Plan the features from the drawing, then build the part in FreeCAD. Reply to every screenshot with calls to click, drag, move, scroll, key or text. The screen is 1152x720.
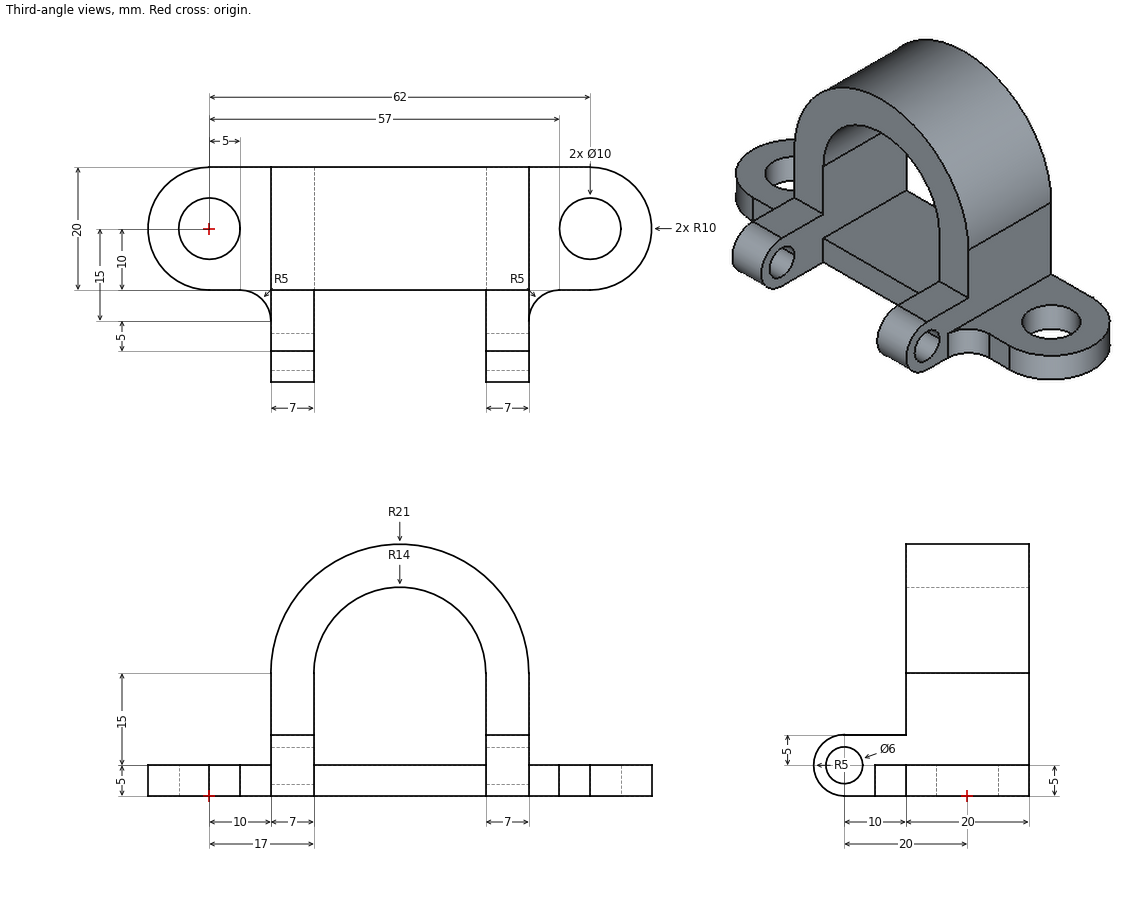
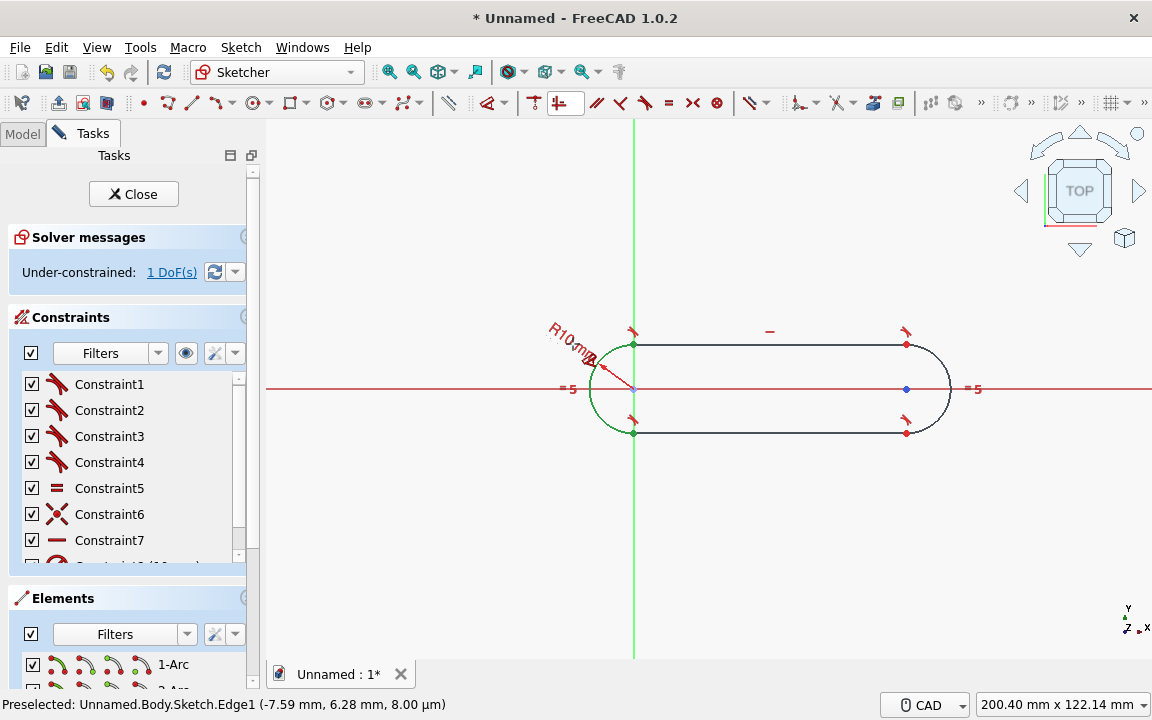
click(716, 345)
click(770, 311)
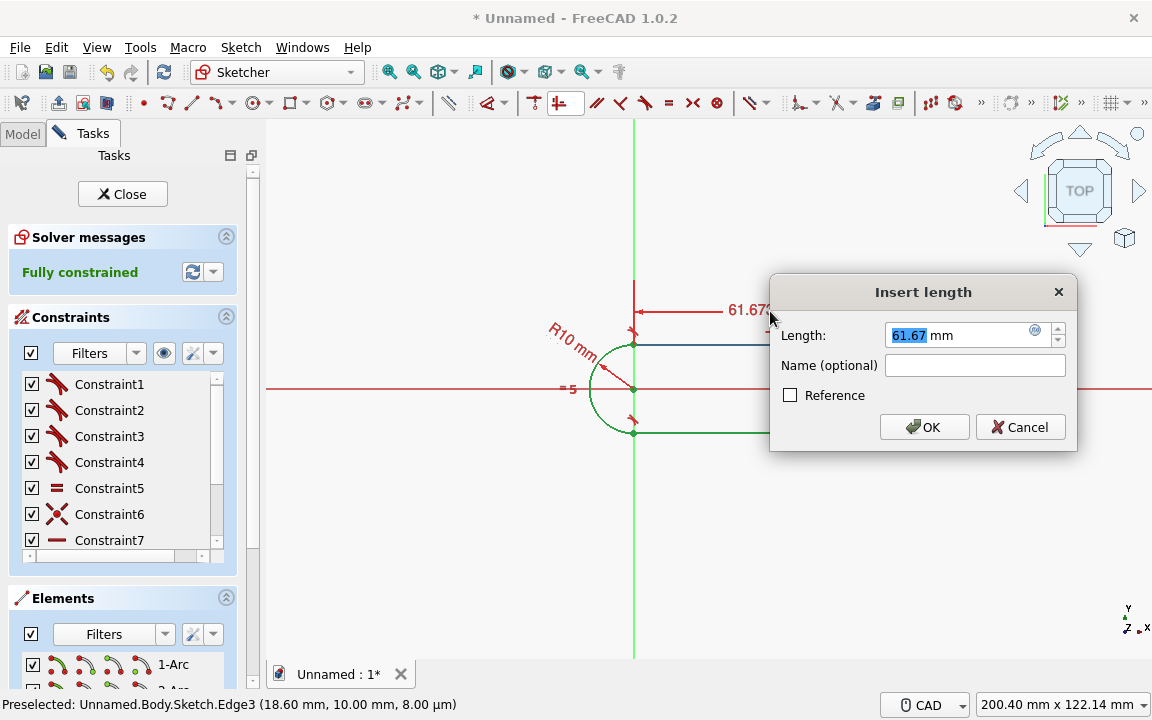
text(62)
key(Return)
key(Escape)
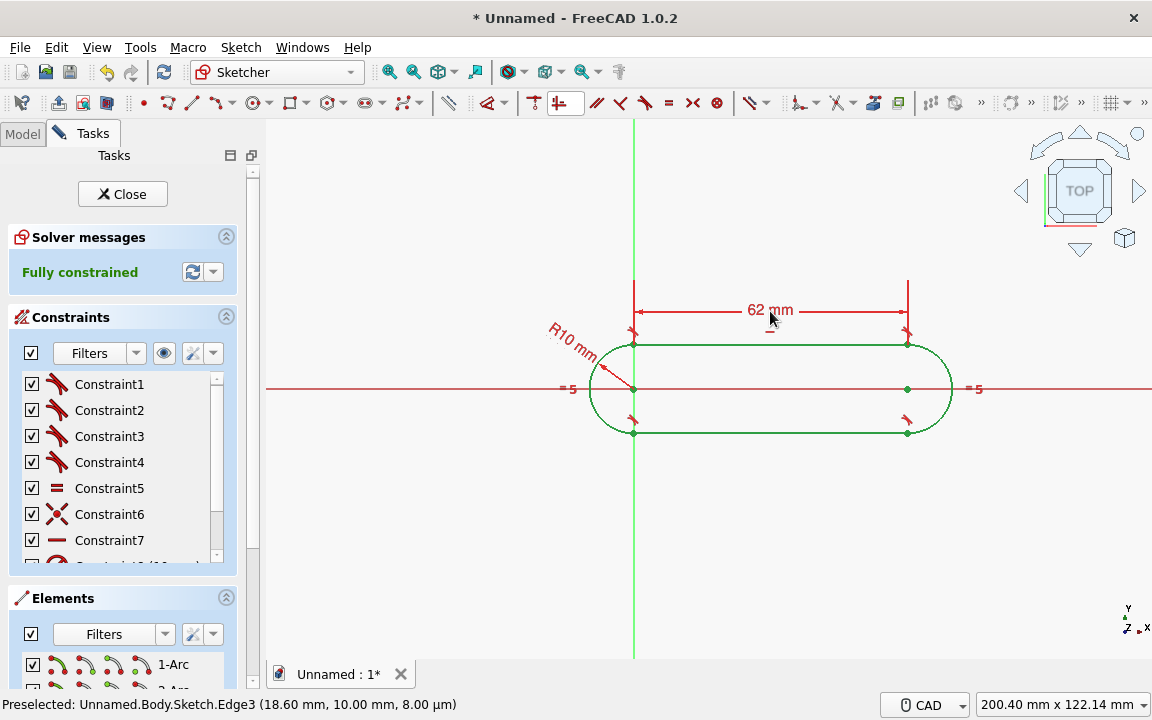
click(123, 194)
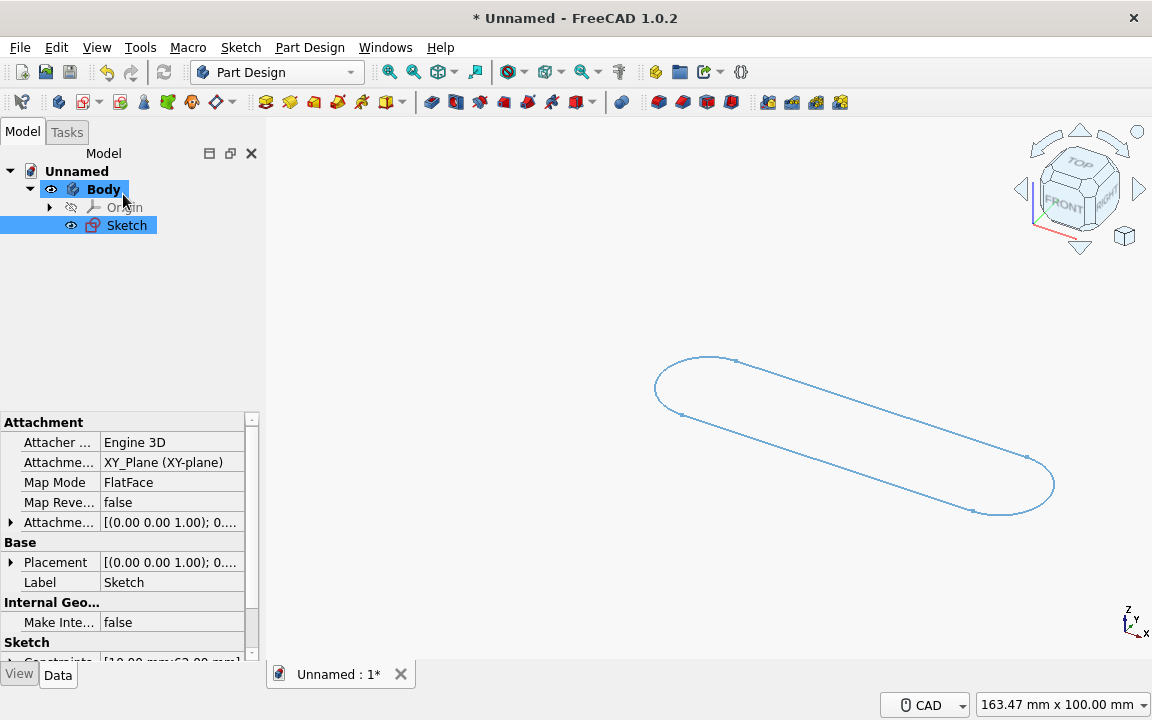
click(266, 102)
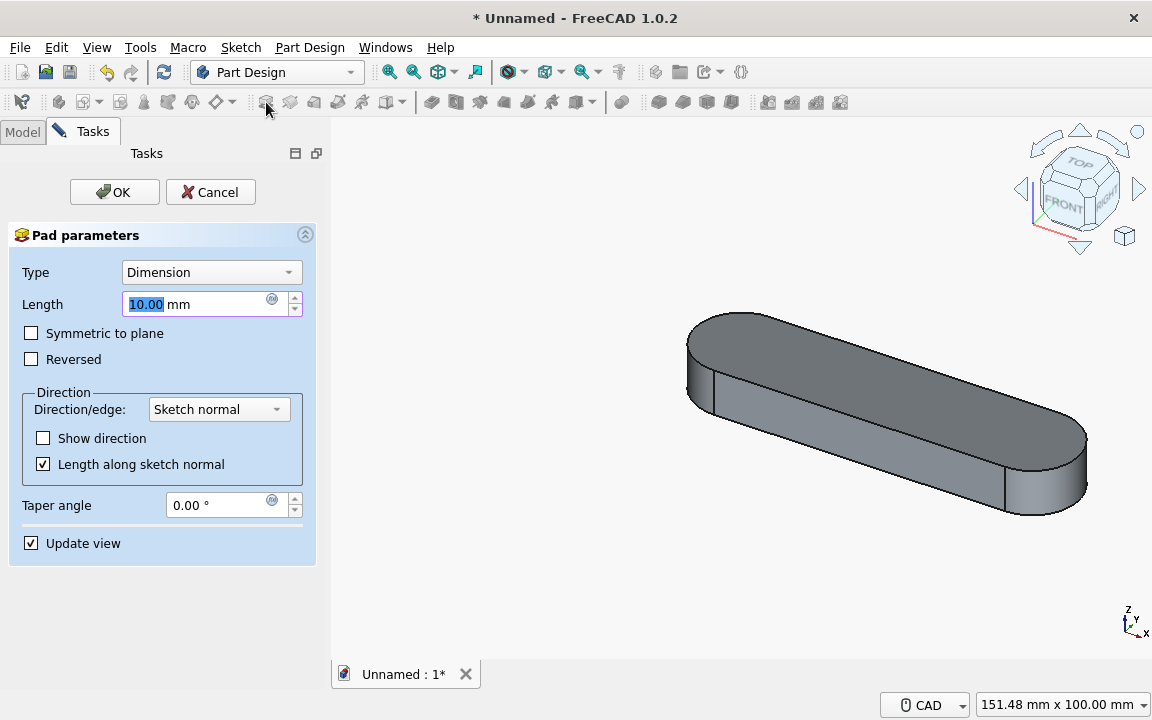
text(5)
key(Tab)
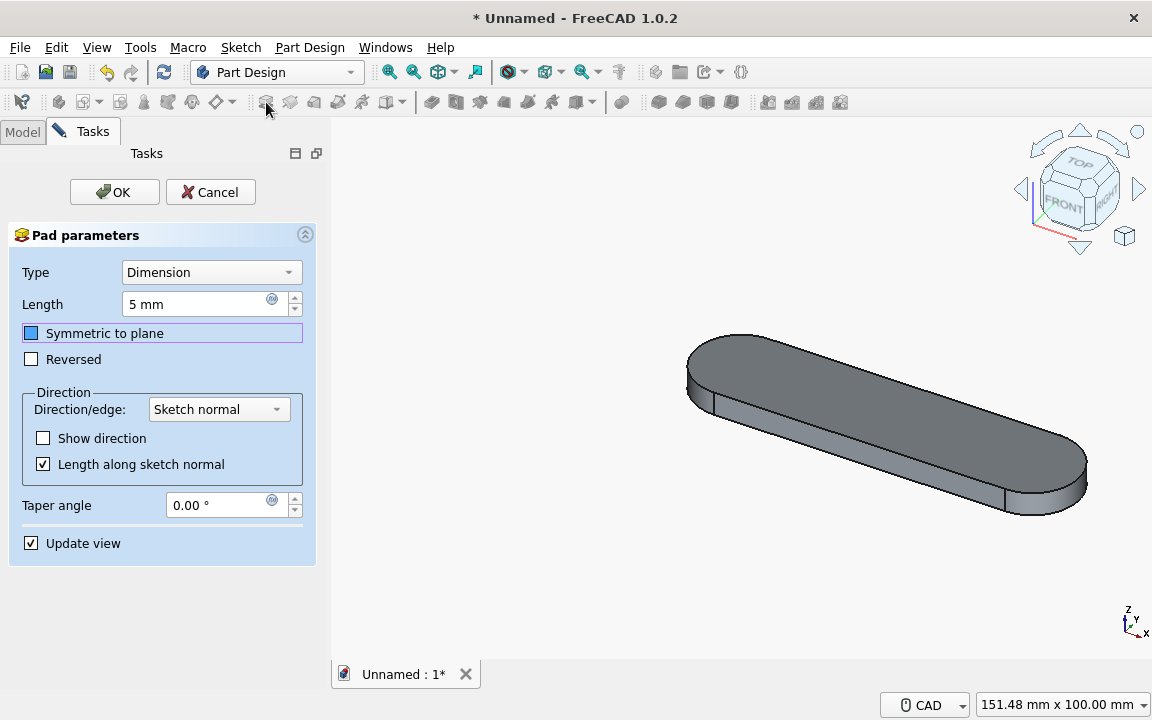
click(115, 192)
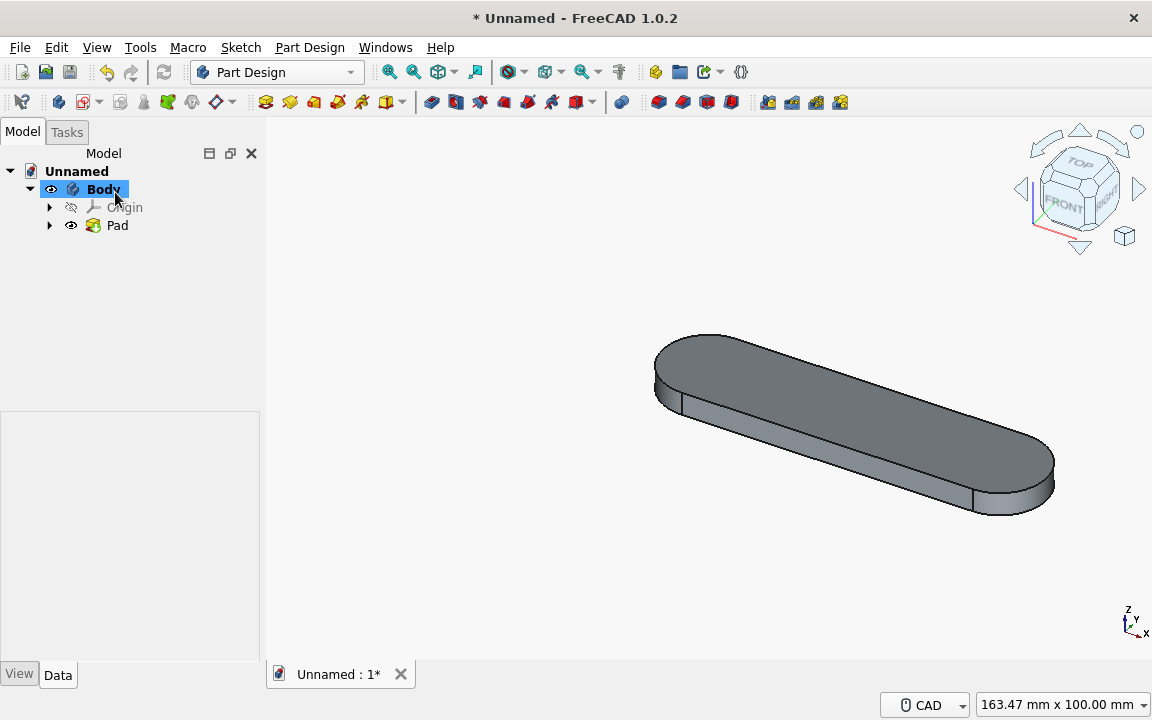
click(952, 492)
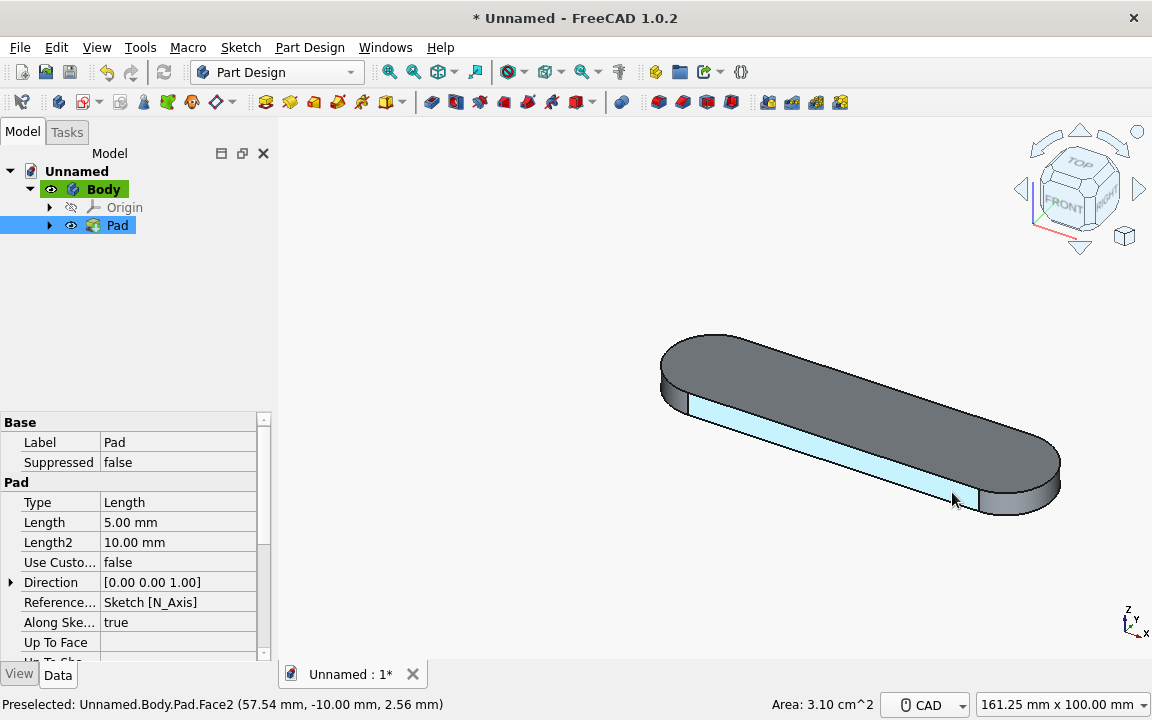
click(84, 102)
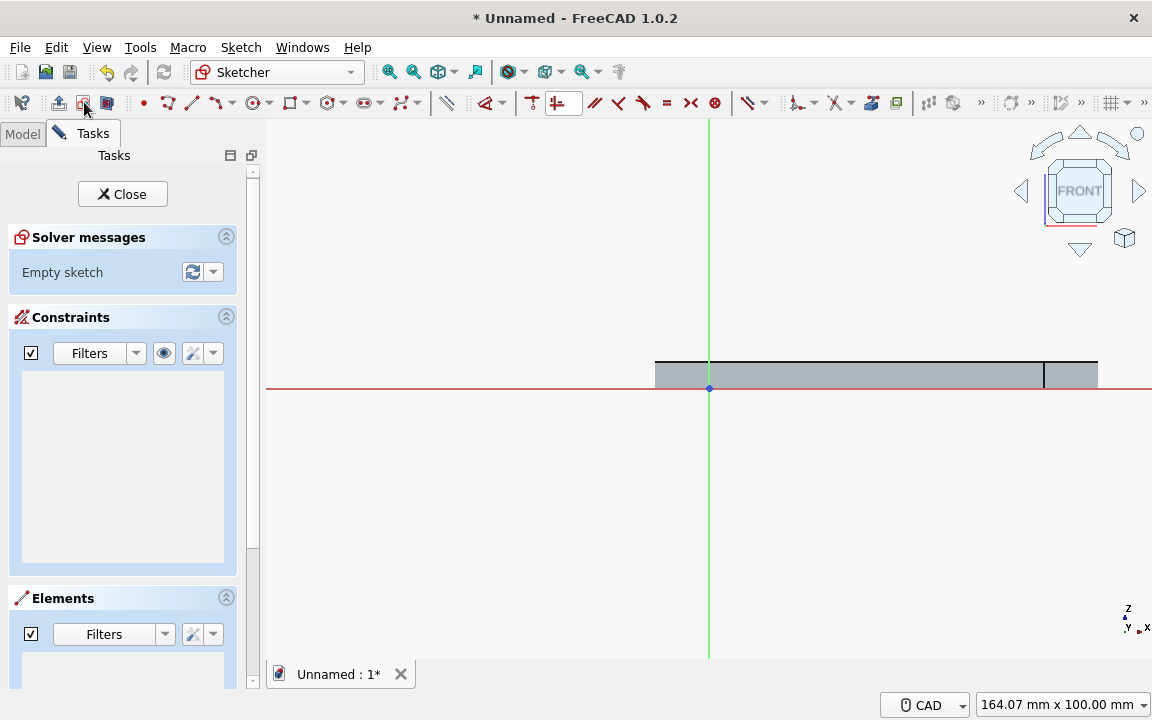
scroll(294, 631, down, 1)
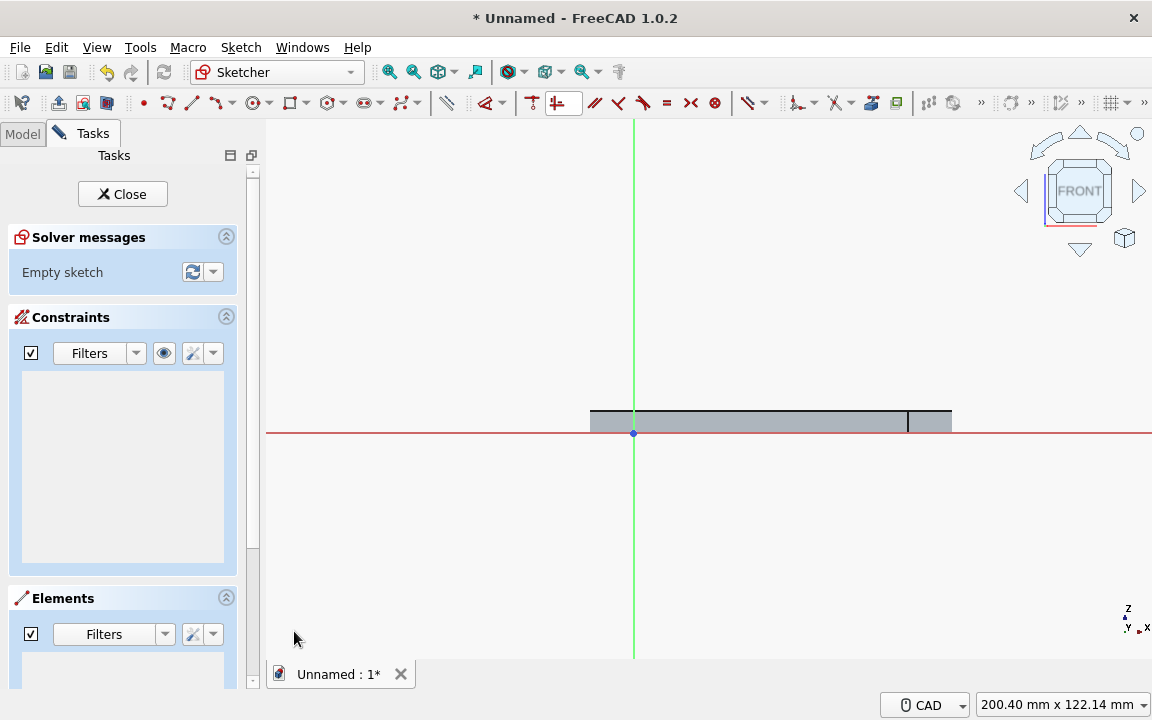
scroll(880, 286, up, 3)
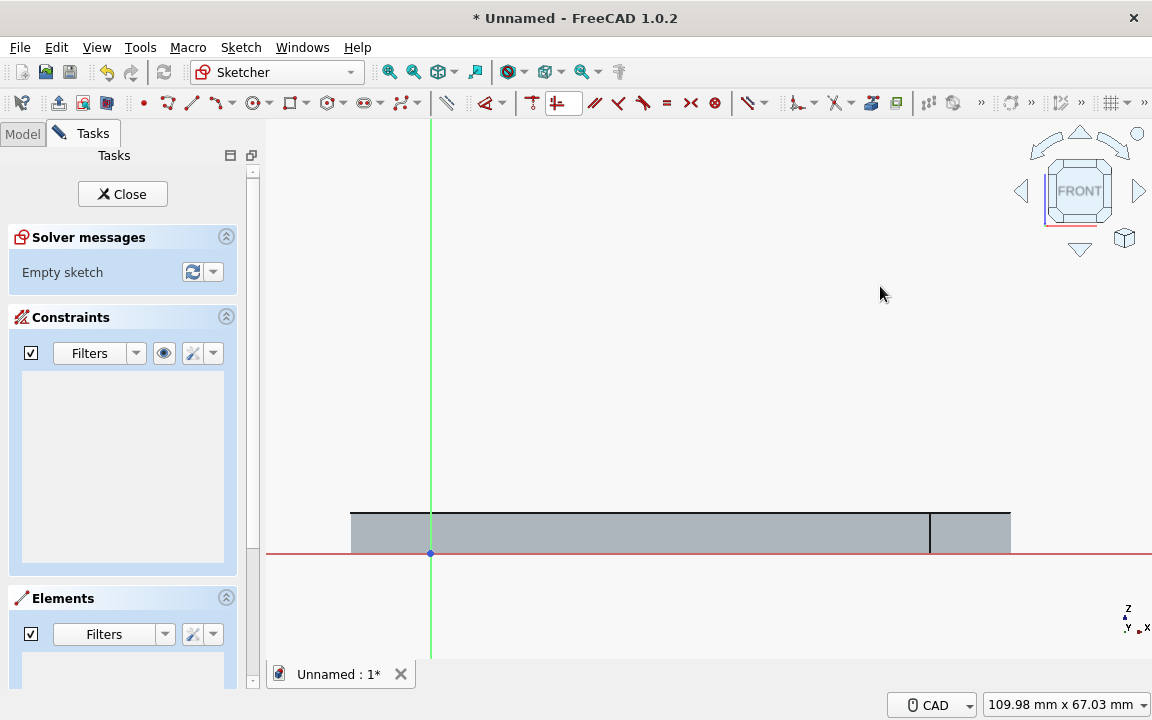
key(g)
key(m)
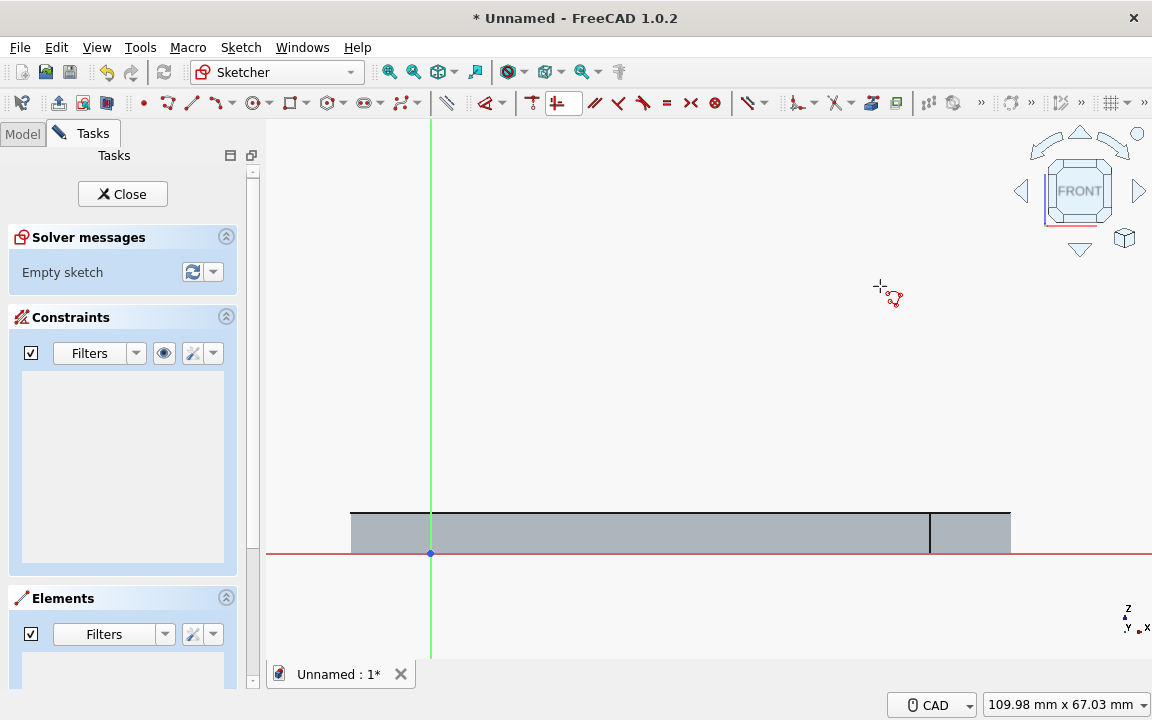
click(511, 393)
click(511, 513)
click(850, 513)
click(850, 393)
right_click(850, 393)